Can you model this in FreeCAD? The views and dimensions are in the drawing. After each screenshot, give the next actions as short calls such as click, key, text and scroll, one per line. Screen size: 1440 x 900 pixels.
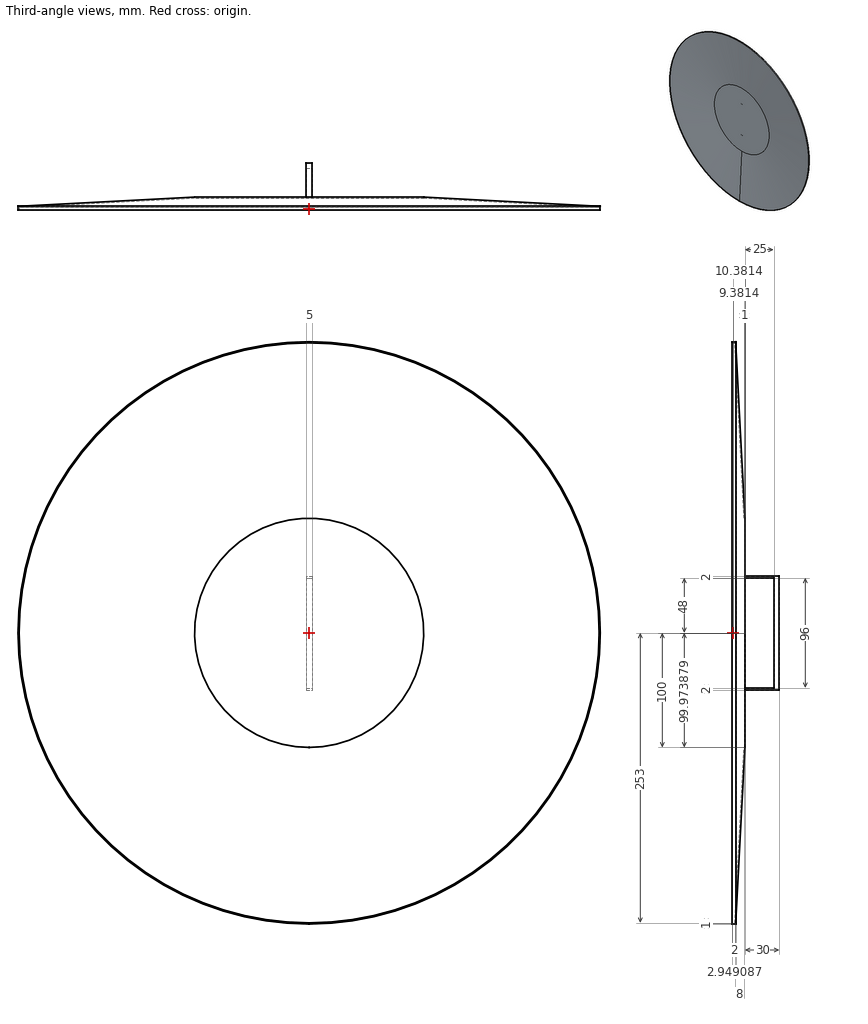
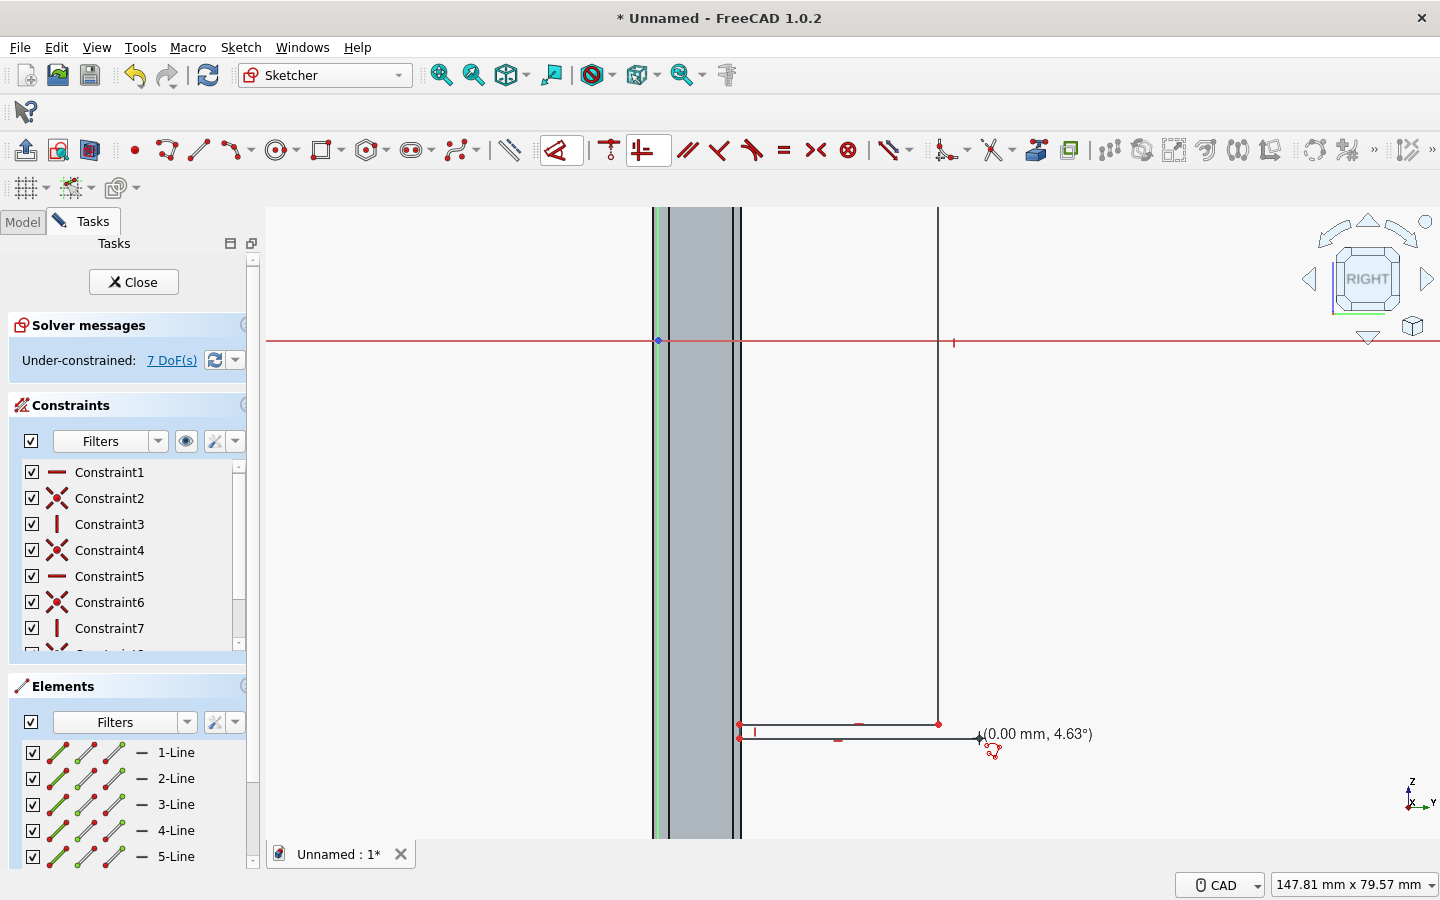
scroll(743, 745, down, 3)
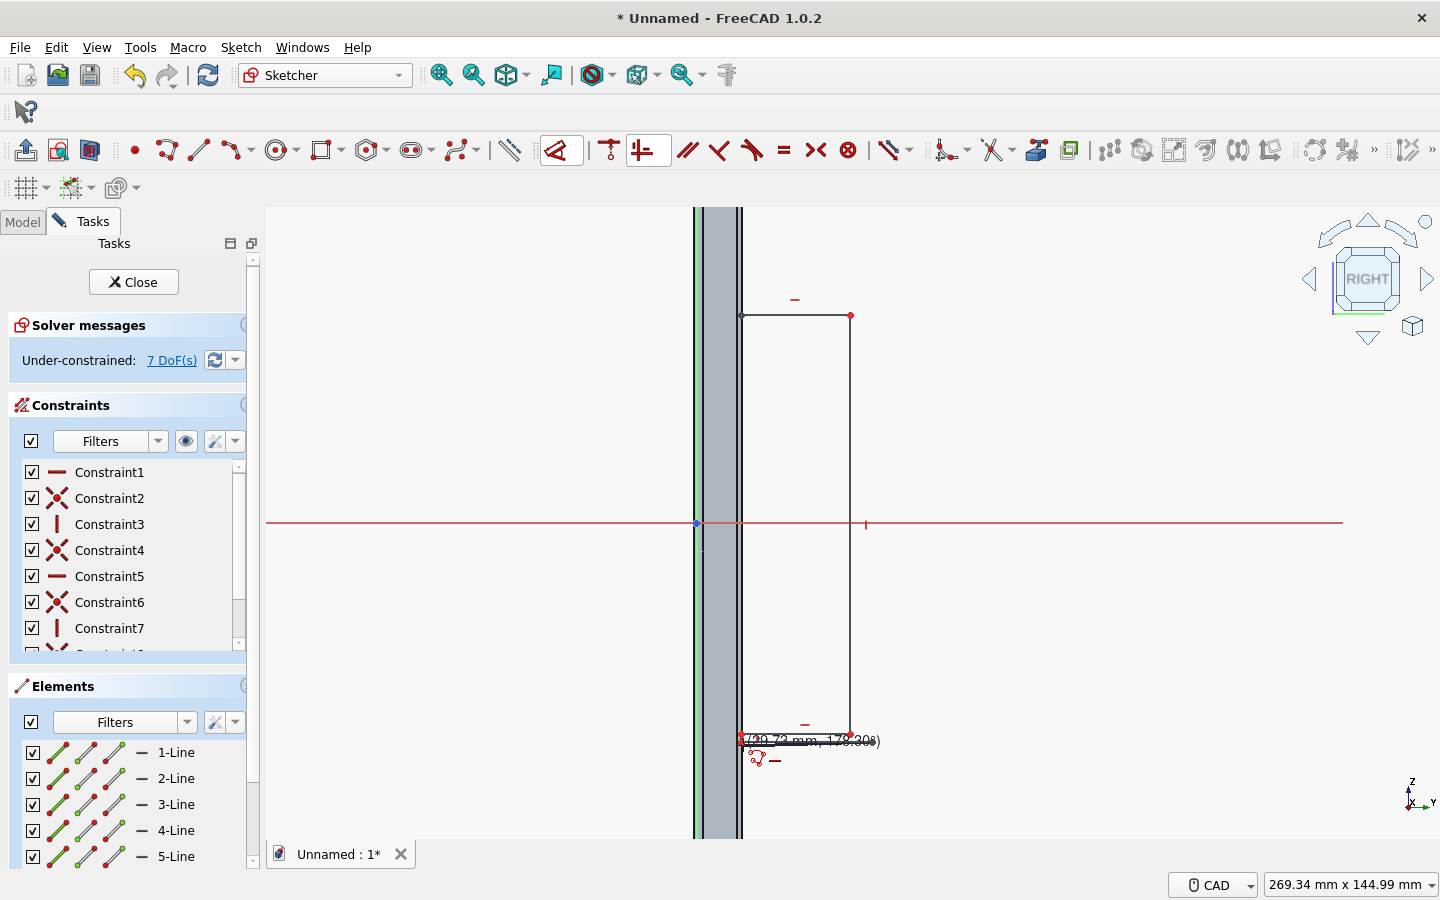
click(873, 306)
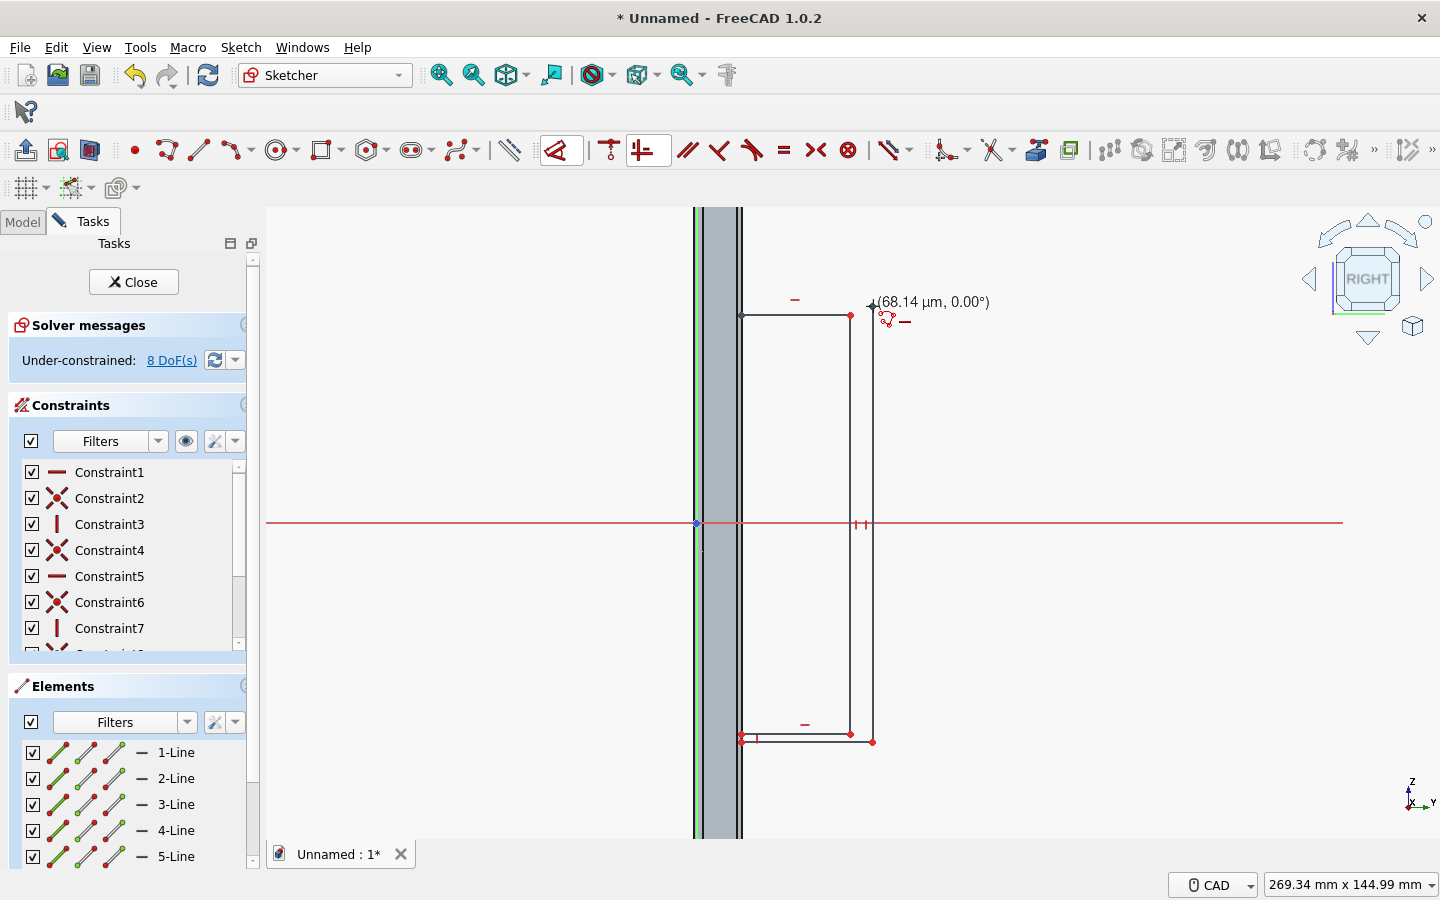
scroll(742, 306, up, 3)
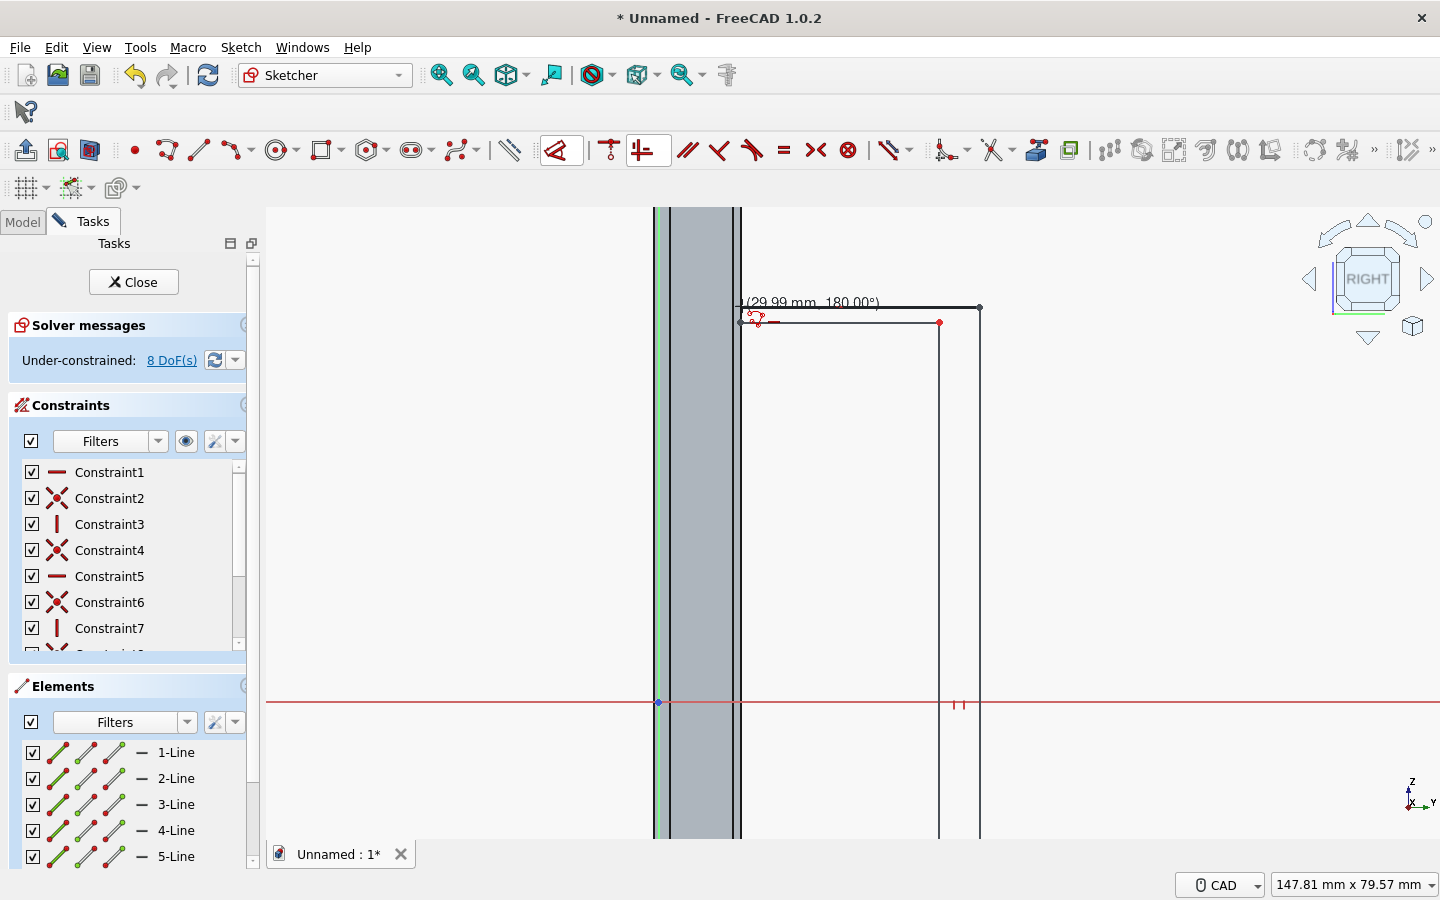
click(741, 306)
click(740, 323)
key(Escape)
key(Escape)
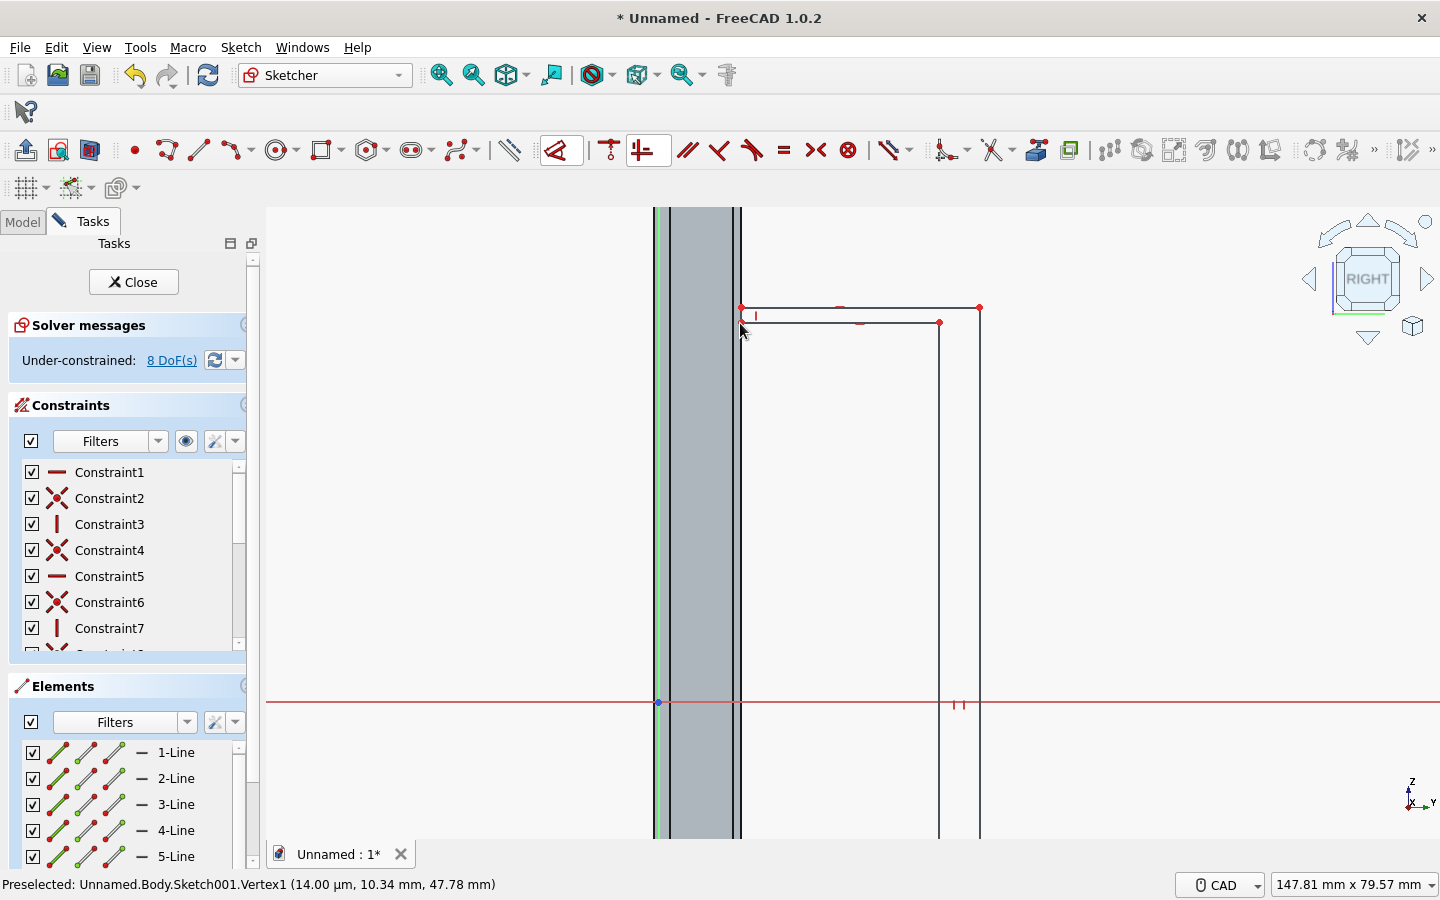
scroll(742, 305, down, 3)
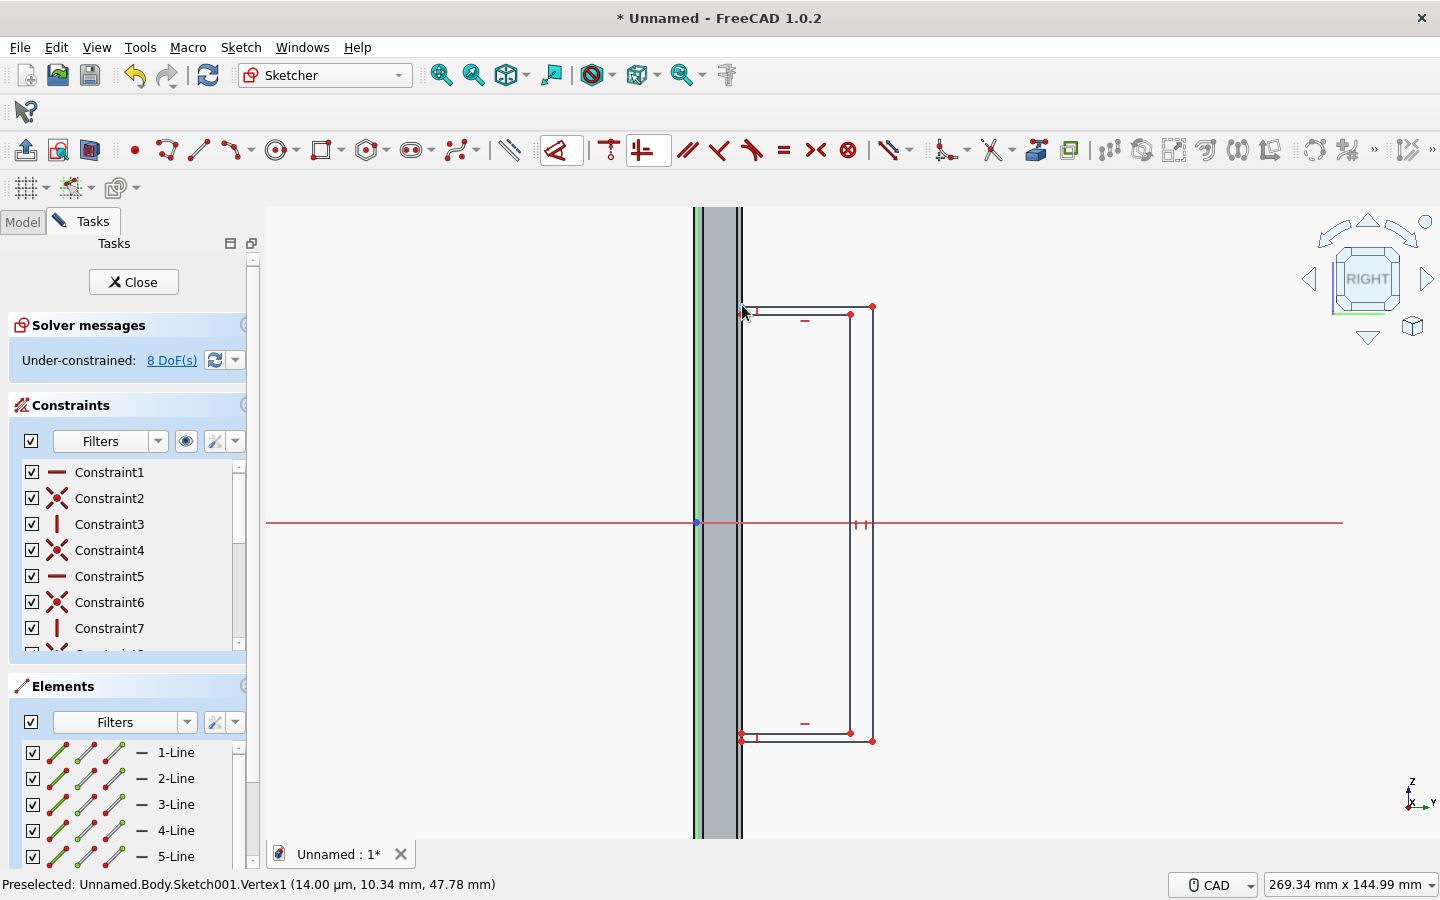
scroll(741, 738, up, 8)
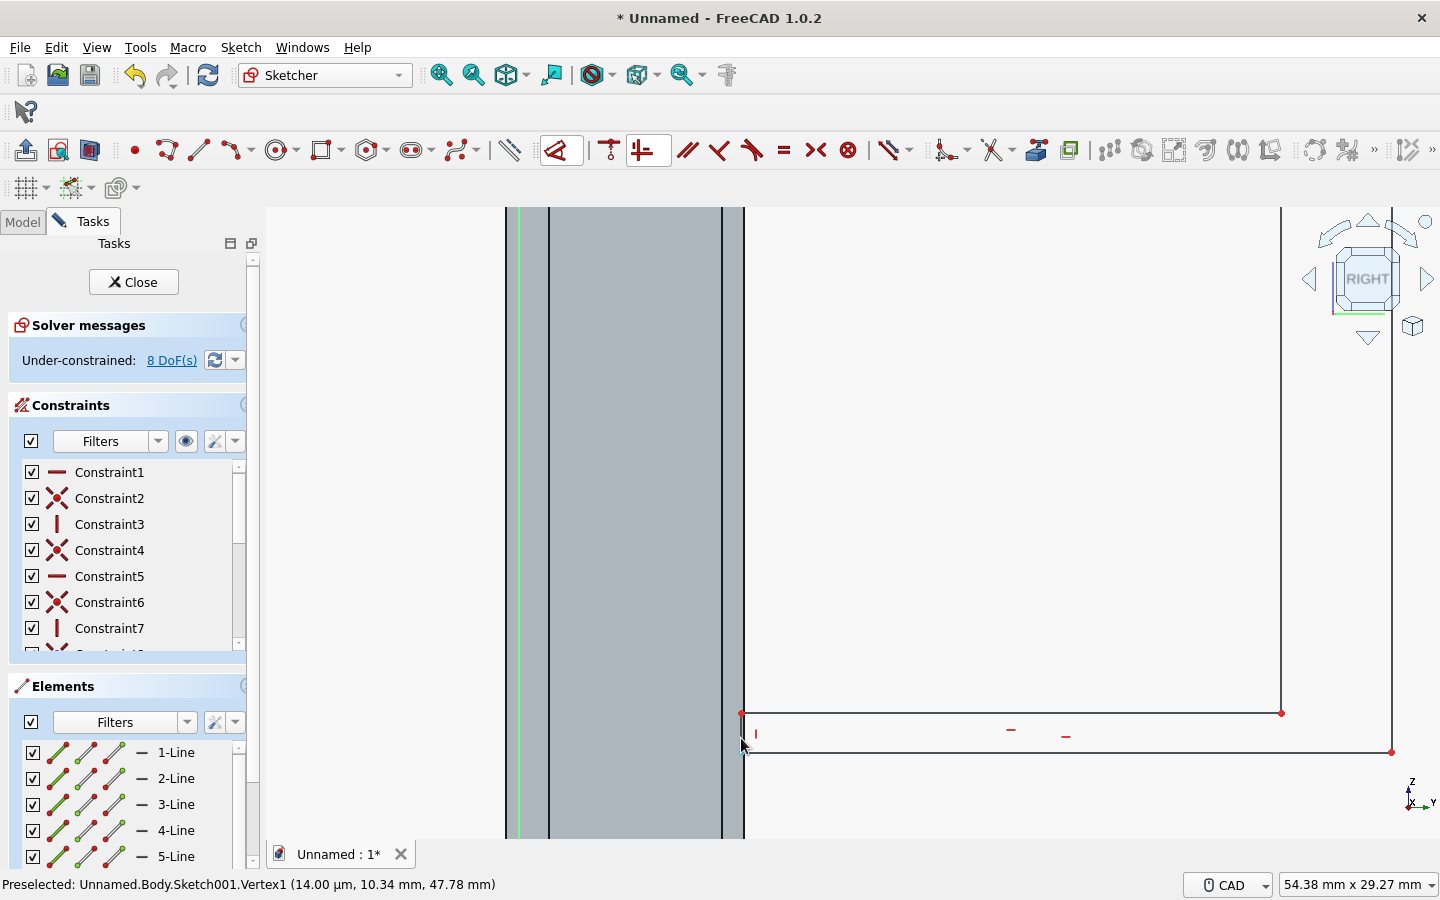
click(741, 733)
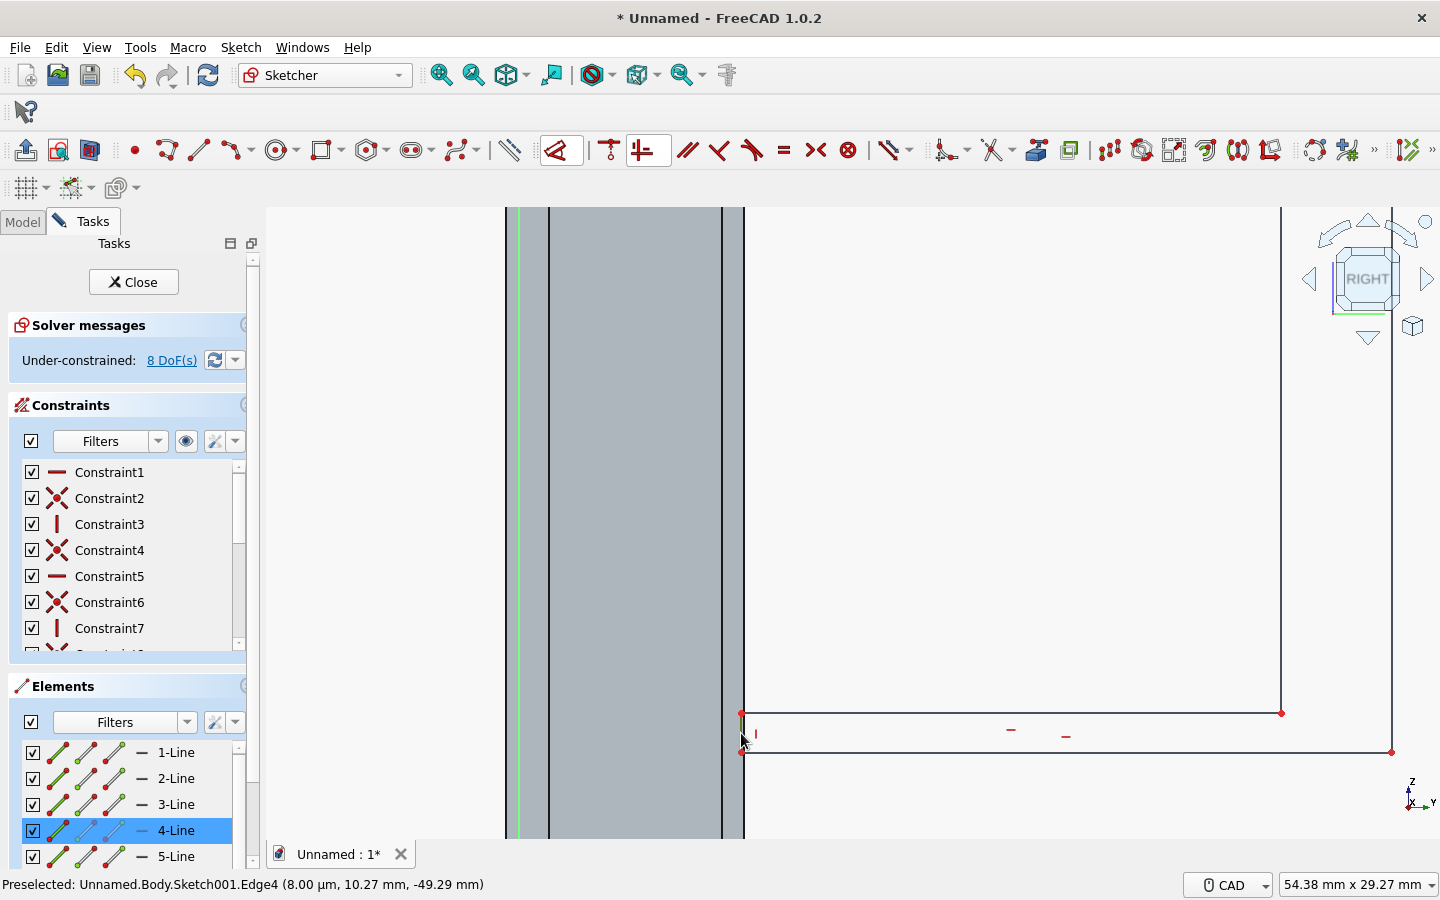
key(i)